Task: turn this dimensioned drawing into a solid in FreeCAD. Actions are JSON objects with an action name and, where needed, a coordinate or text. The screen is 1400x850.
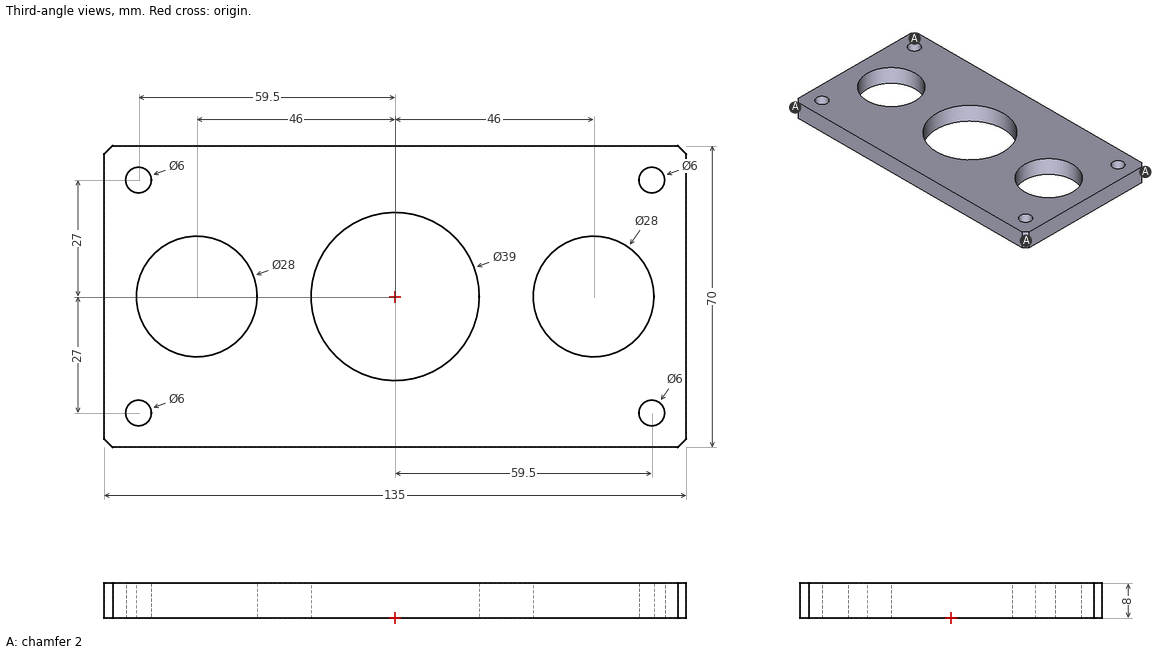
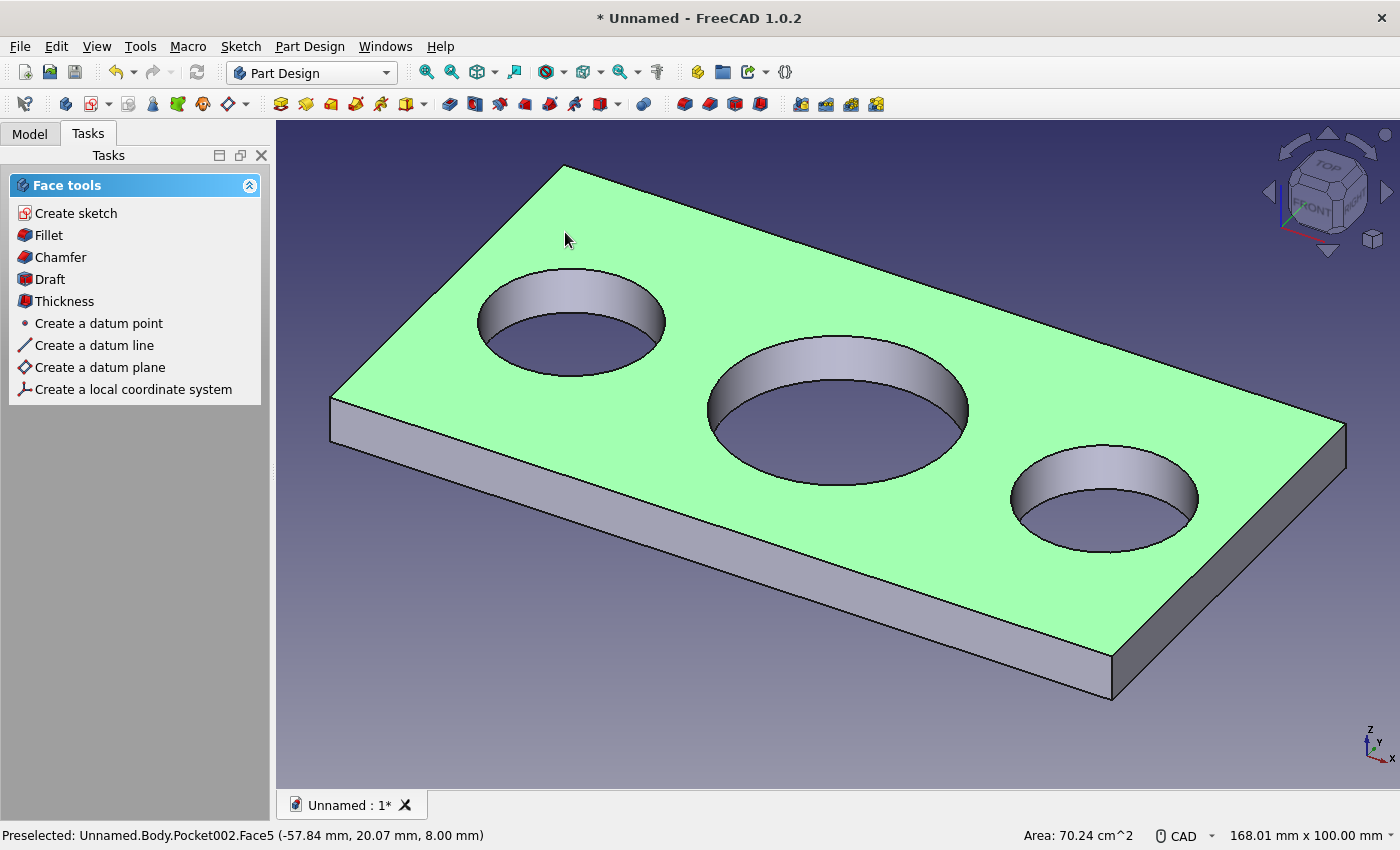
{"action": "left_click", "coordinate": [90, 104]}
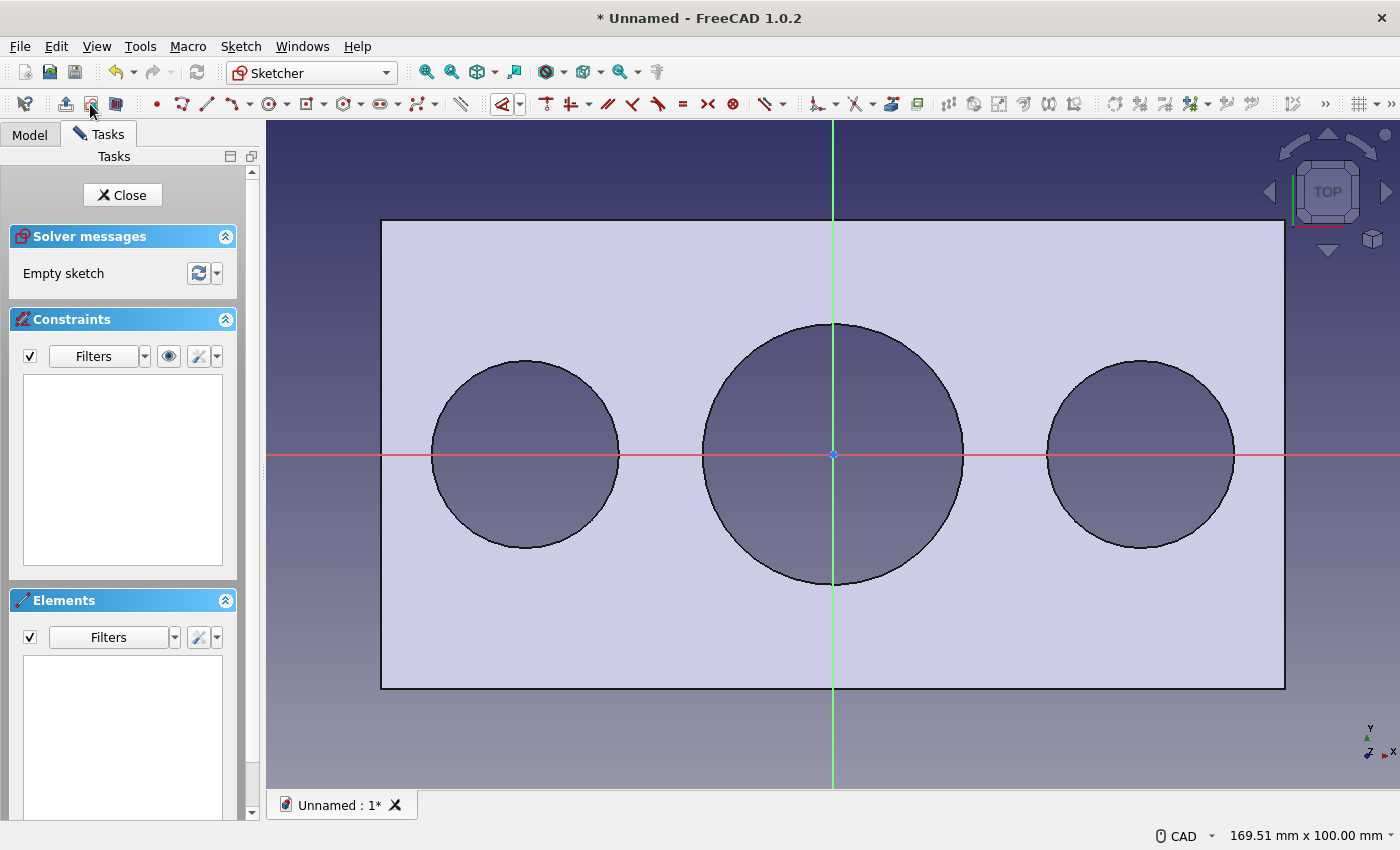
{"action": "scroll", "coordinate": [402, 256], "scroll_direction": "up", "scroll_amount": 12}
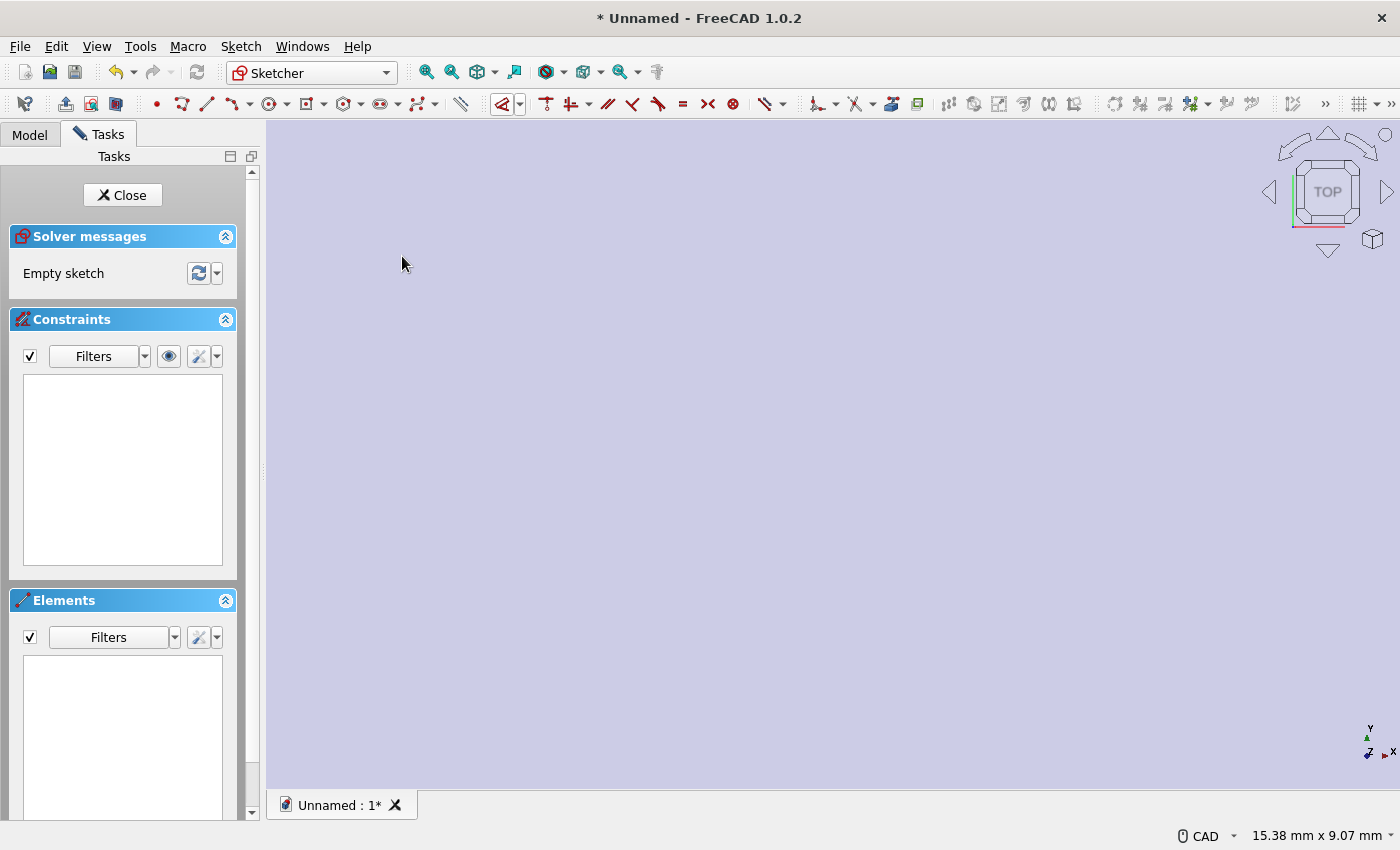
{"action": "key", "text": "g c"}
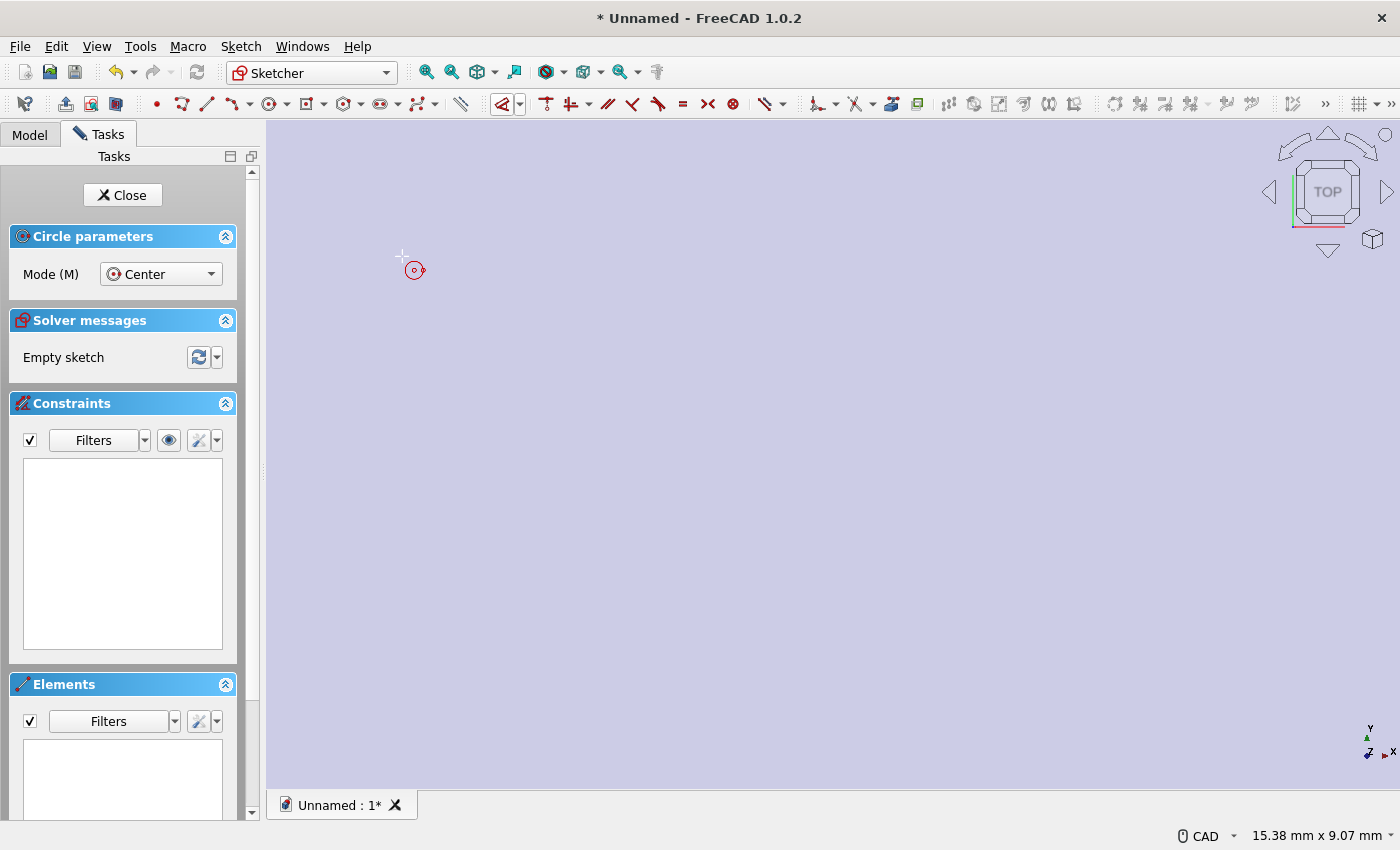
{"action": "left_click", "coordinate": [764, 451]}
{"action": "left_click", "coordinate": [920, 295]}
{"action": "key", "text": "Escape"}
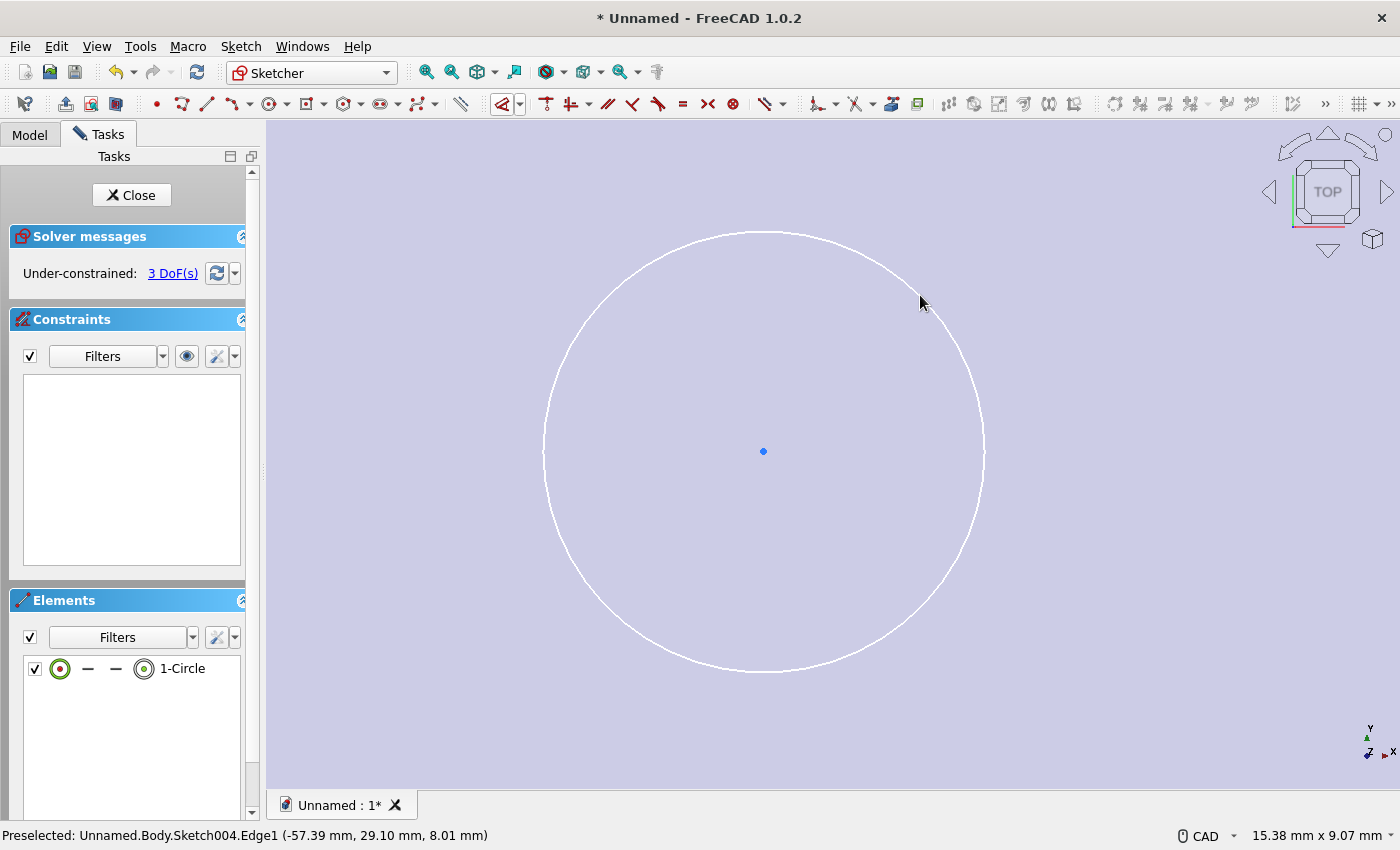
{"action": "left_click", "coordinate": [920, 296]}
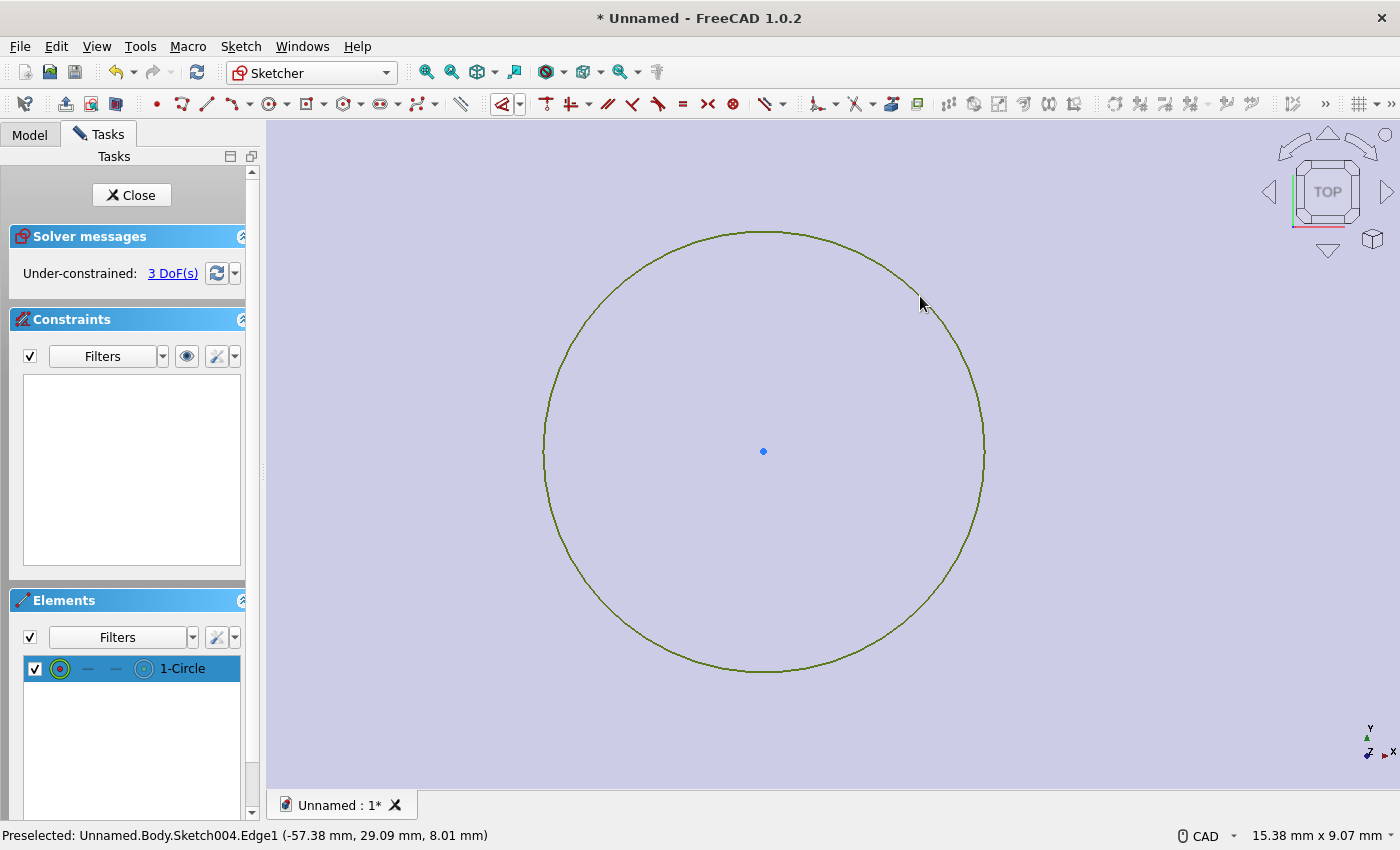
{"action": "left_click", "coordinate": [520, 104]}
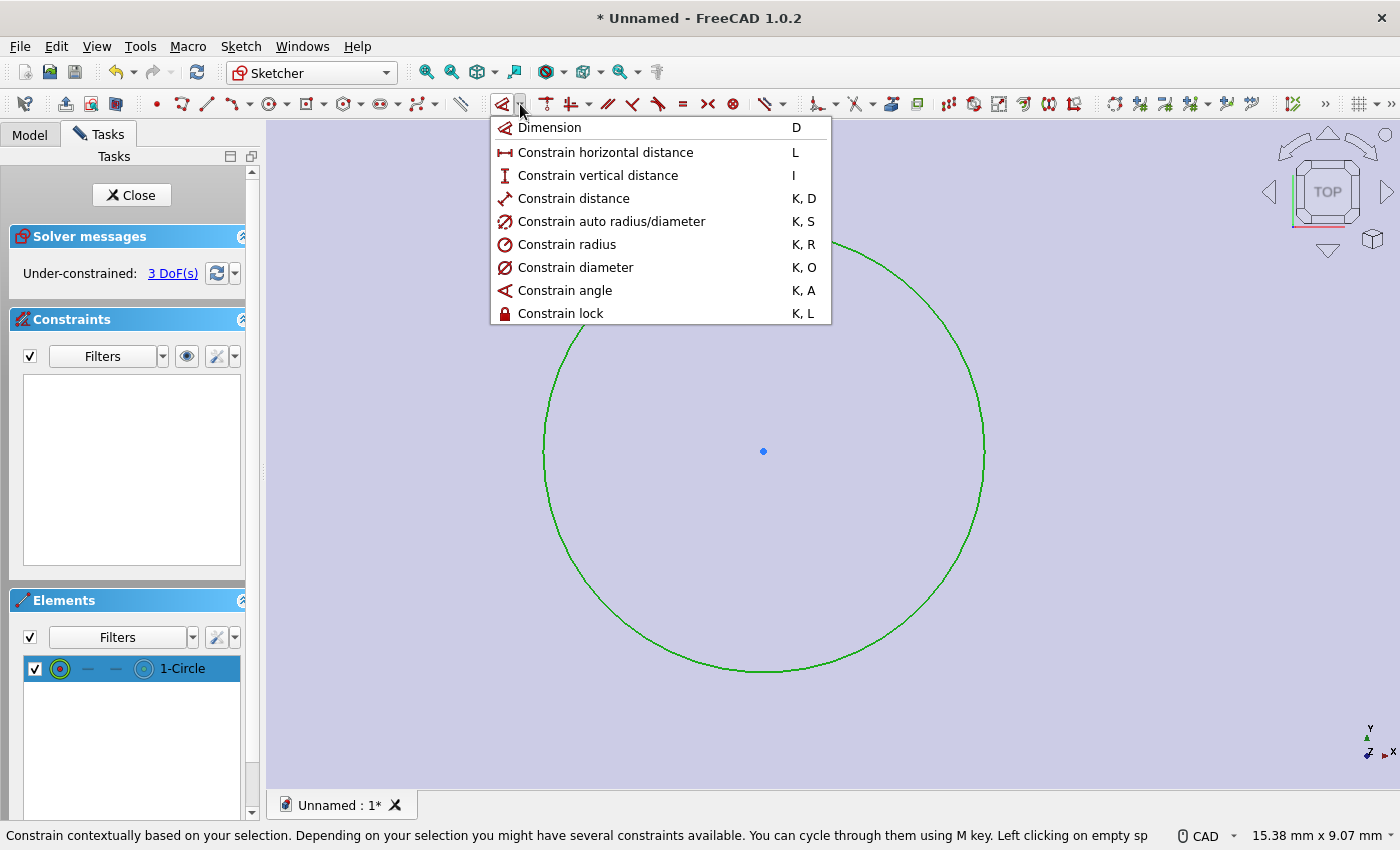
{"action": "left_click", "coordinate": [661, 268]}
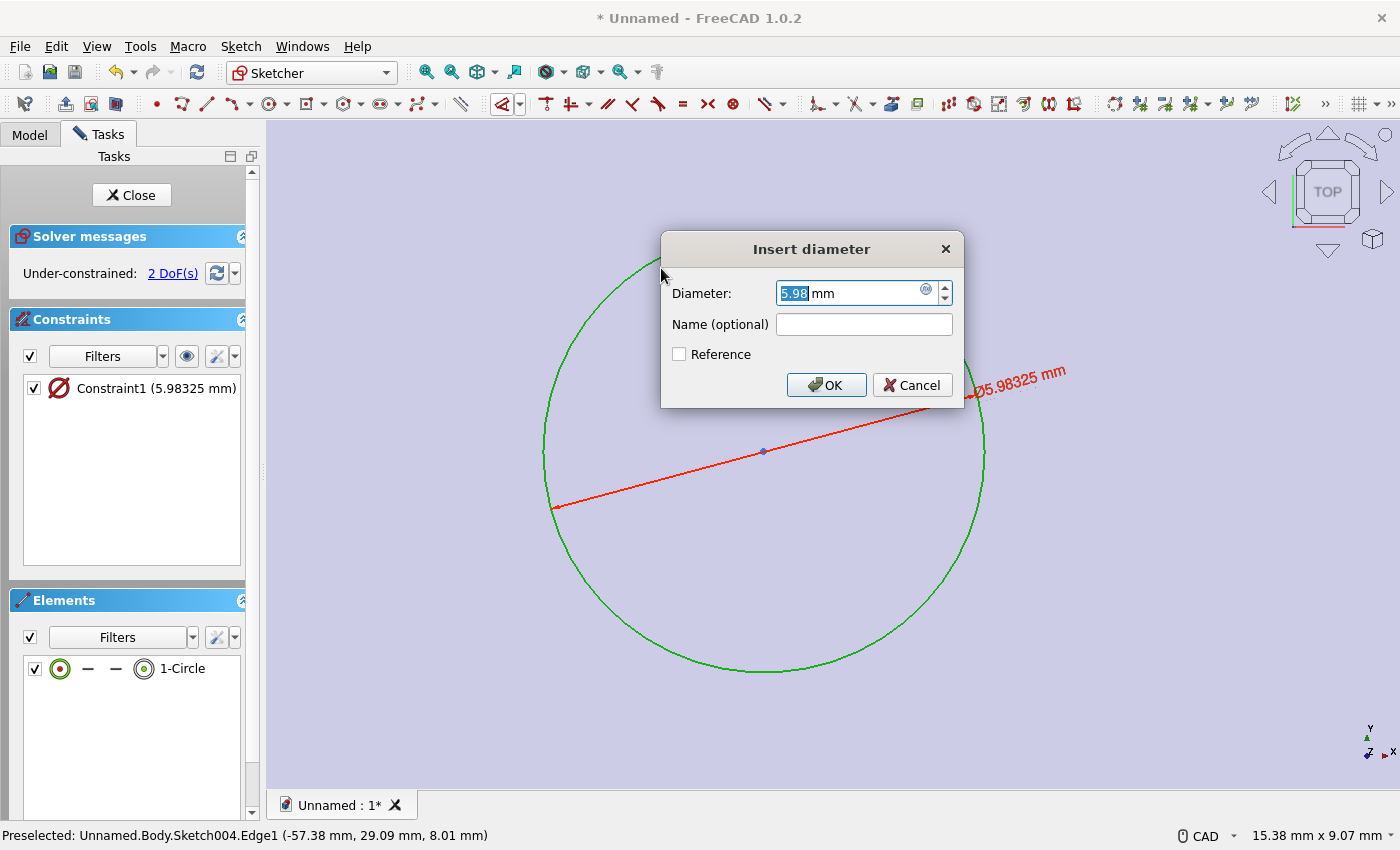
{"action": "type", "text": "6"}
{"action": "key", "text": "Return"}